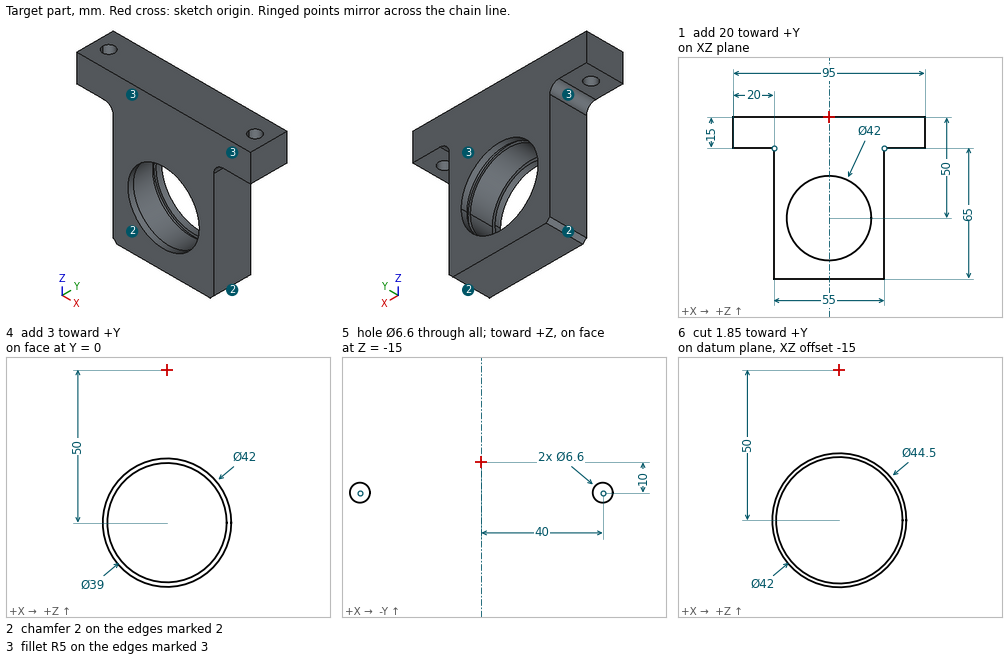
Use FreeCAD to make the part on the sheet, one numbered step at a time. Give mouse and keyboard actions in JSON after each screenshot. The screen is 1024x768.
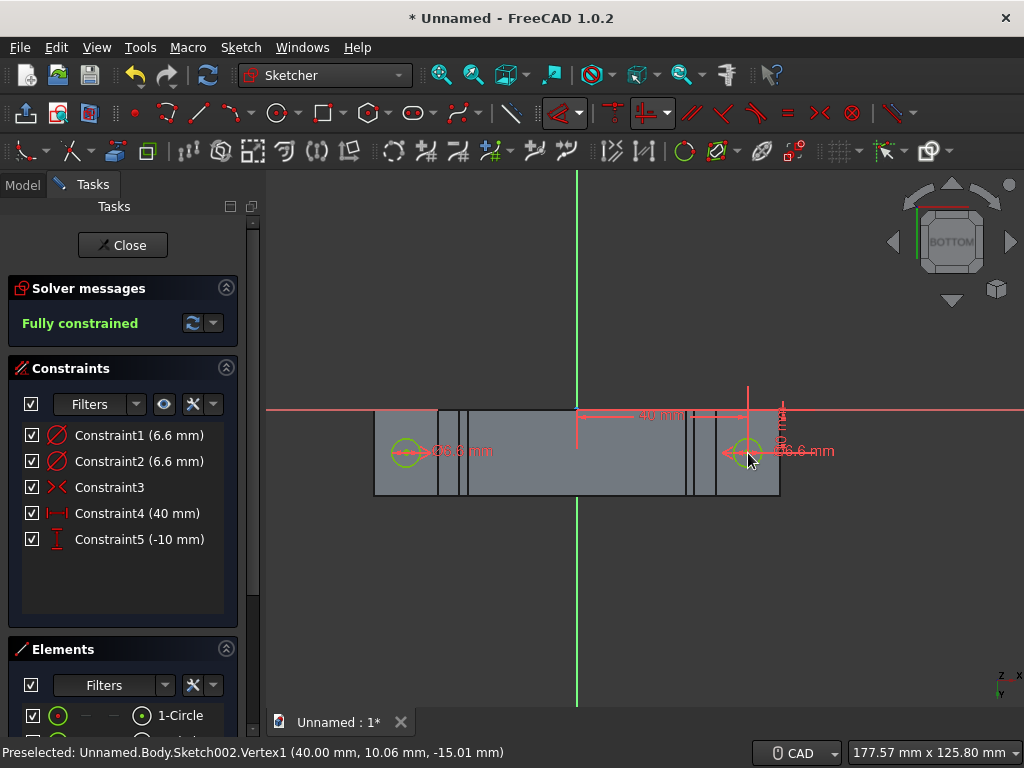
{"action": "left_click", "coordinate": [123, 245]}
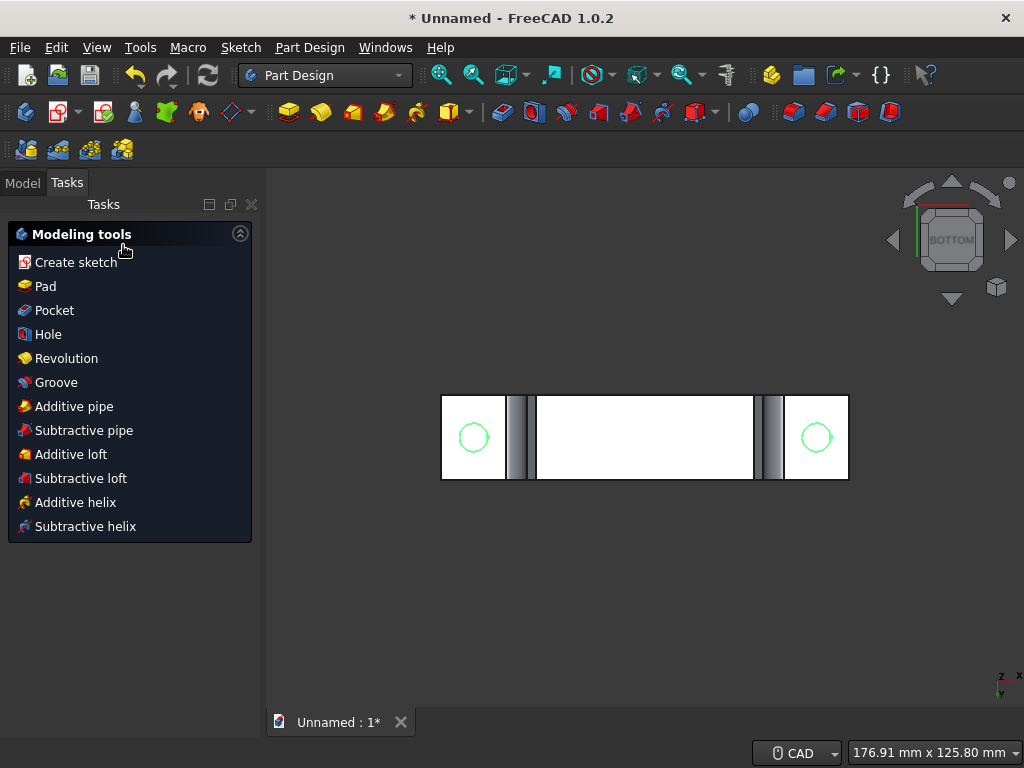
{"action": "left_click", "coordinate": [536, 112]}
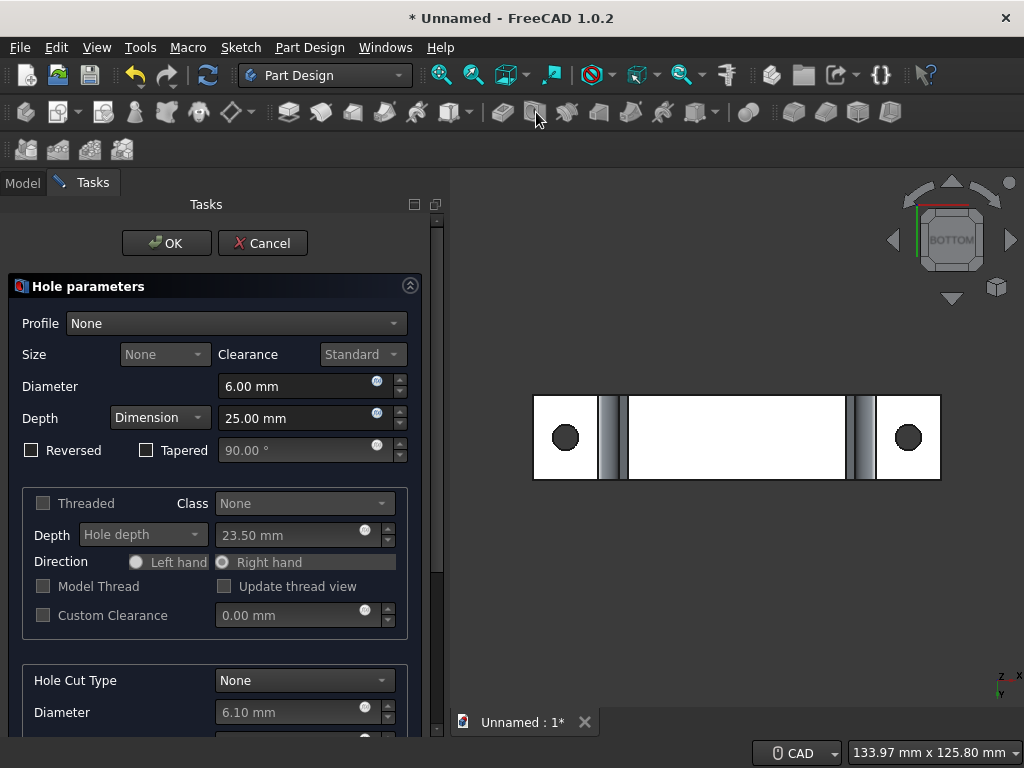
{"action": "triple_click", "coordinate": [305, 386]}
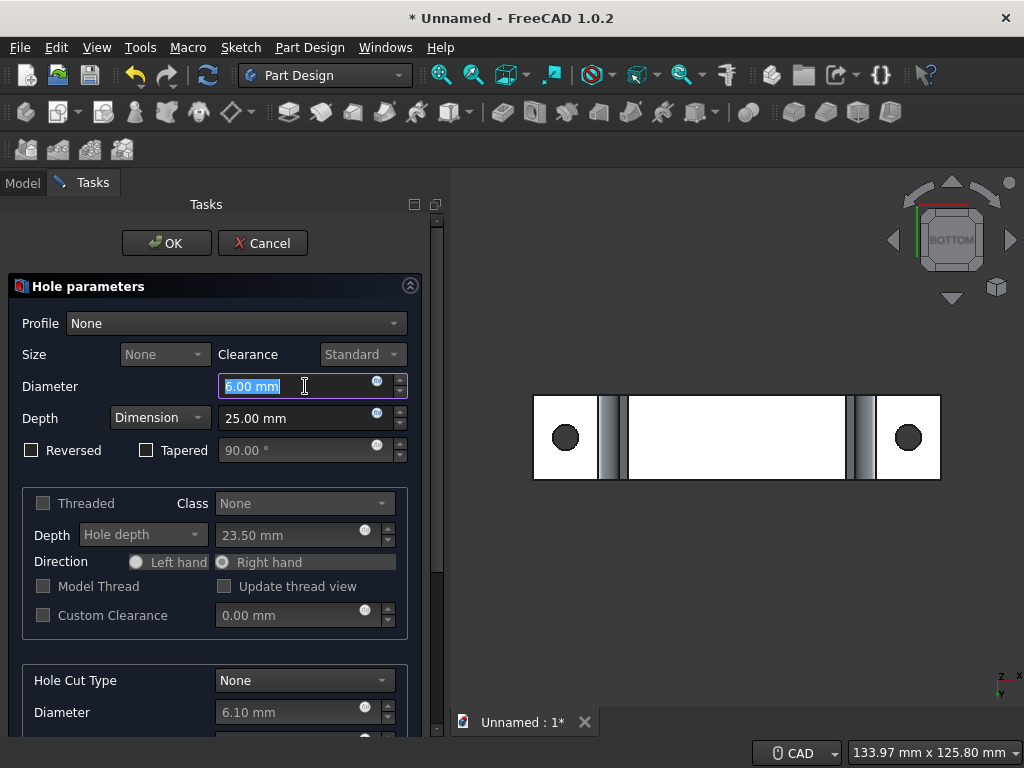
{"action": "type", "text": "6.6"}
{"action": "key", "text": "Tab"}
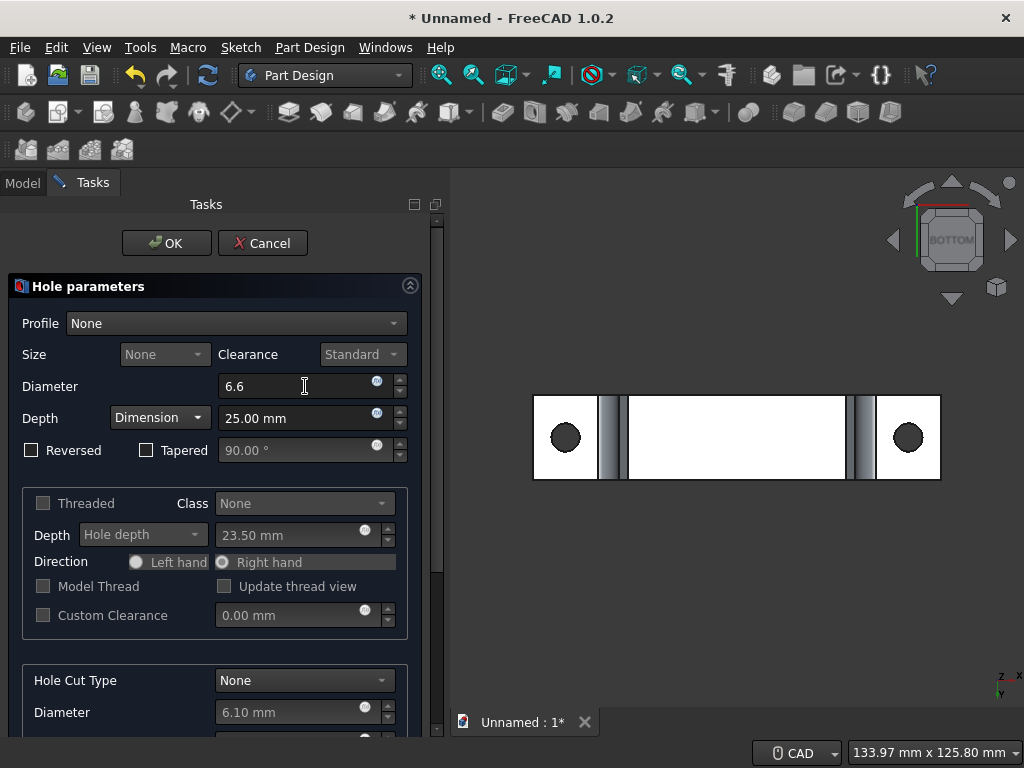
{"action": "left_click", "coordinate": [161, 418]}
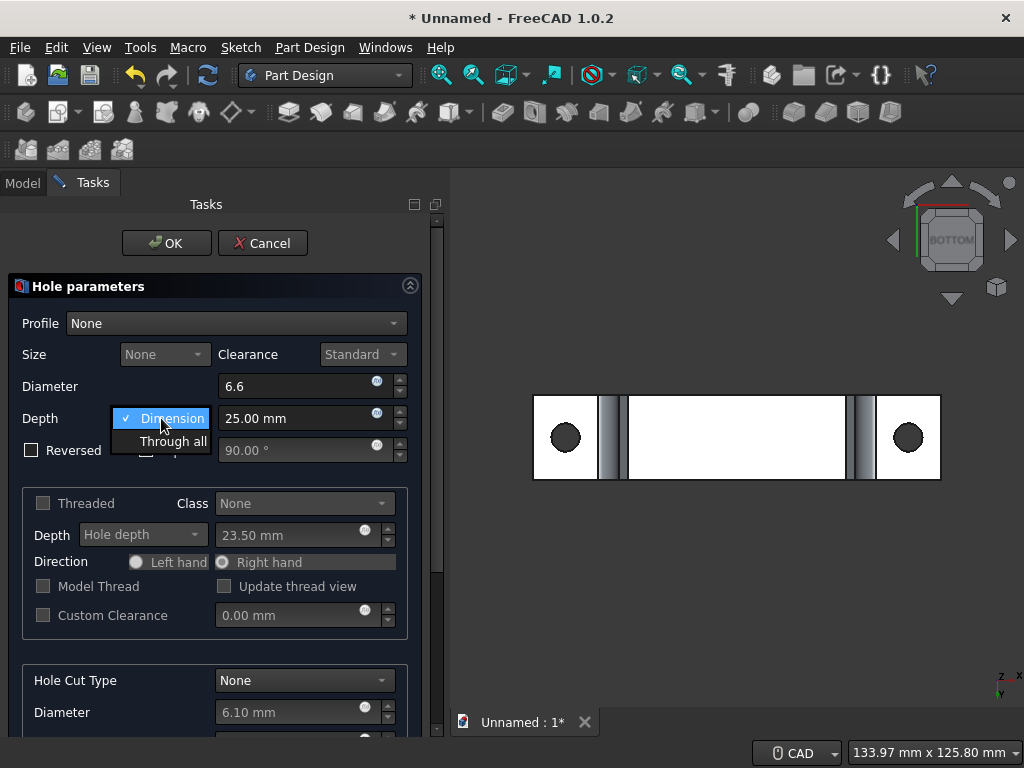
{"action": "left_click", "coordinate": [160, 442]}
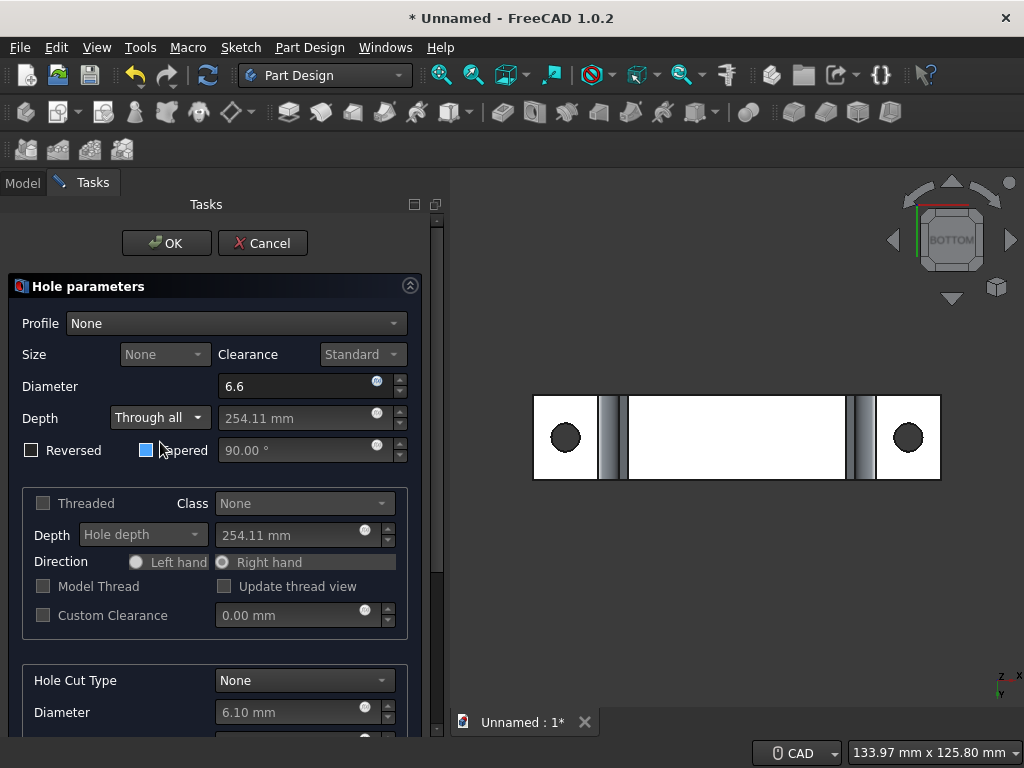
{"action": "left_click", "coordinate": [167, 243]}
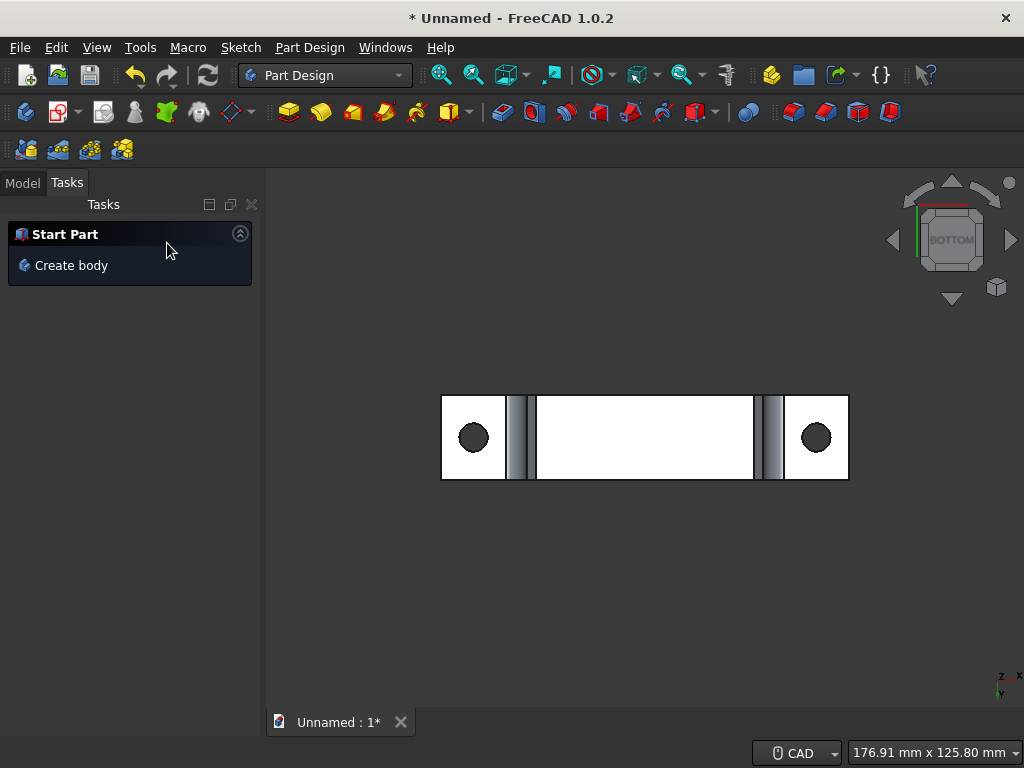
{"action": "left_click", "coordinate": [23, 182]}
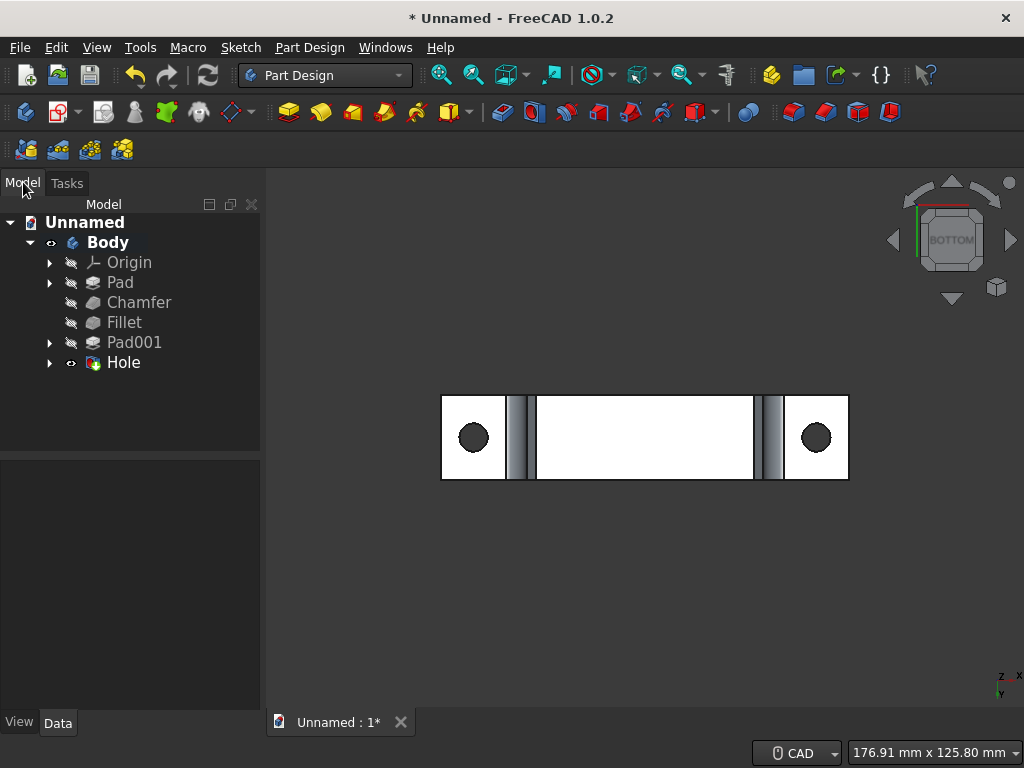
{"action": "left_click", "coordinate": [50, 263]}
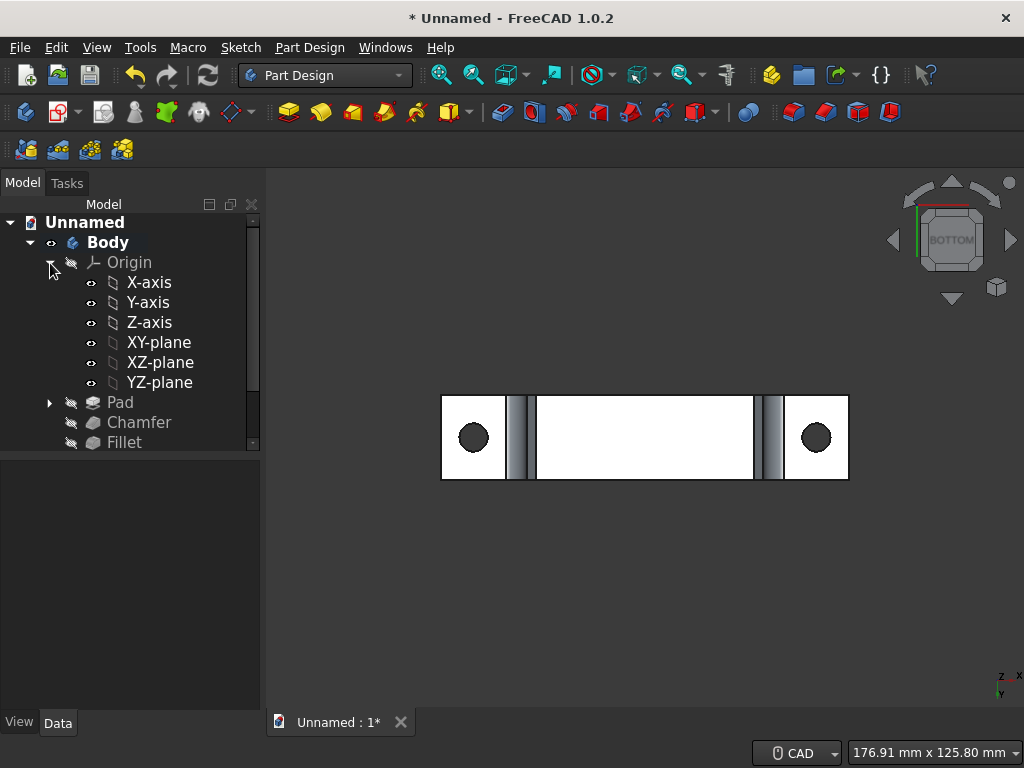
{"action": "left_click", "coordinate": [136, 363]}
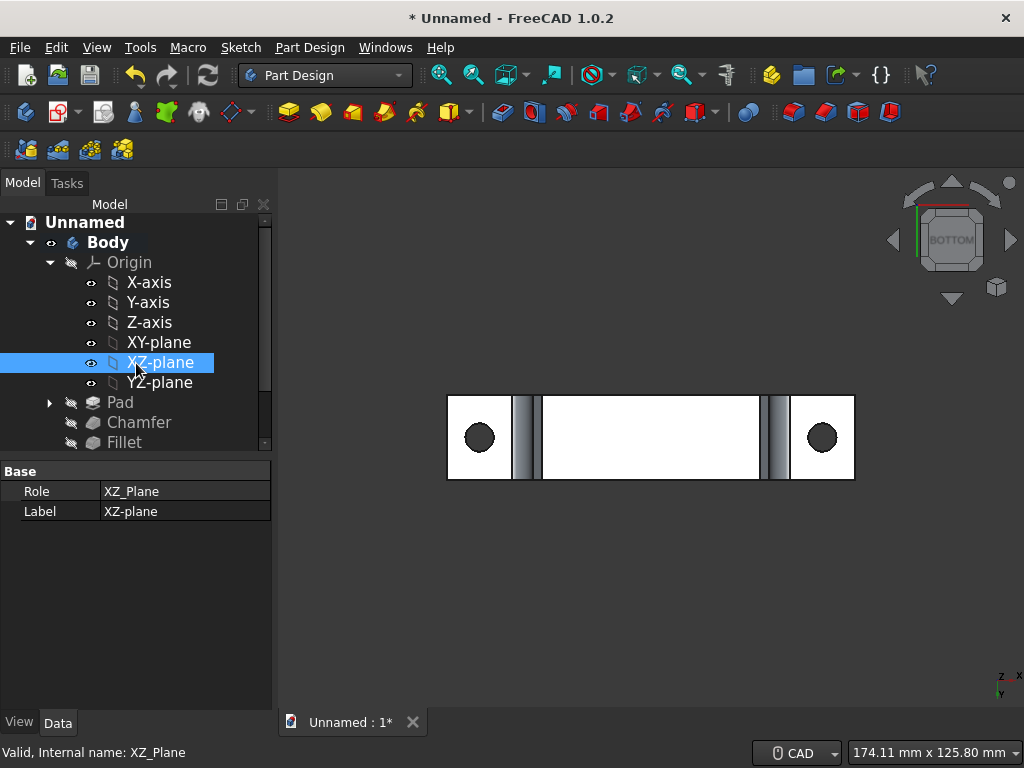
{"action": "left_click", "coordinate": [232, 112]}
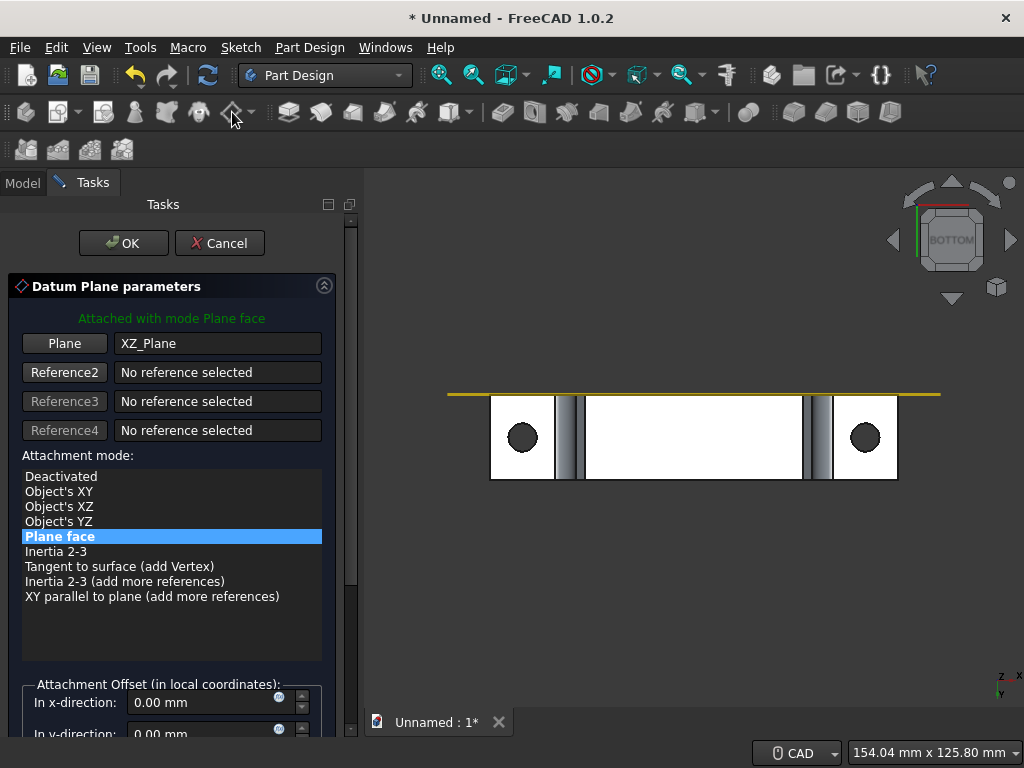
{"action": "scroll", "coordinate": [351, 475], "scroll_direction": "down", "scroll_amount": 2}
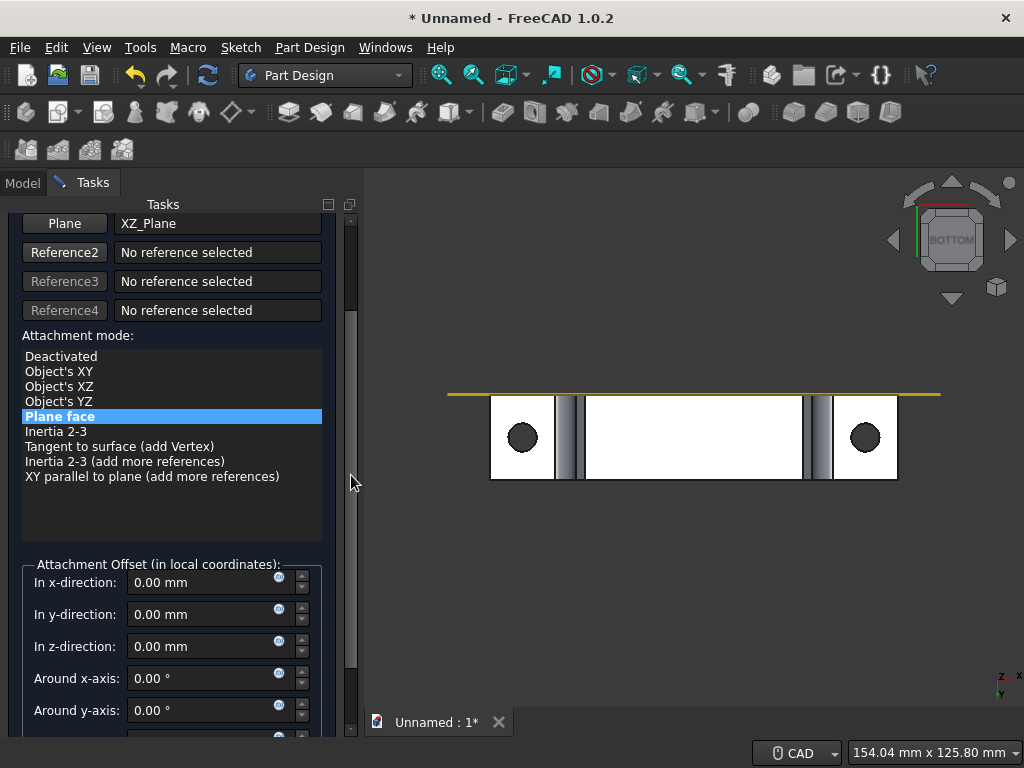
{"action": "triple_click", "coordinate": [210, 646]}